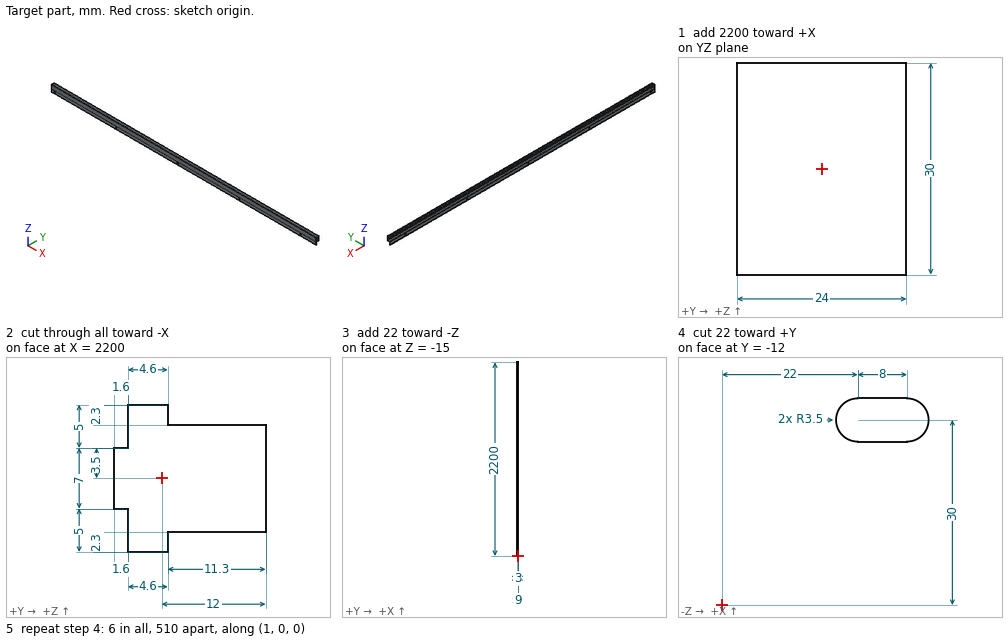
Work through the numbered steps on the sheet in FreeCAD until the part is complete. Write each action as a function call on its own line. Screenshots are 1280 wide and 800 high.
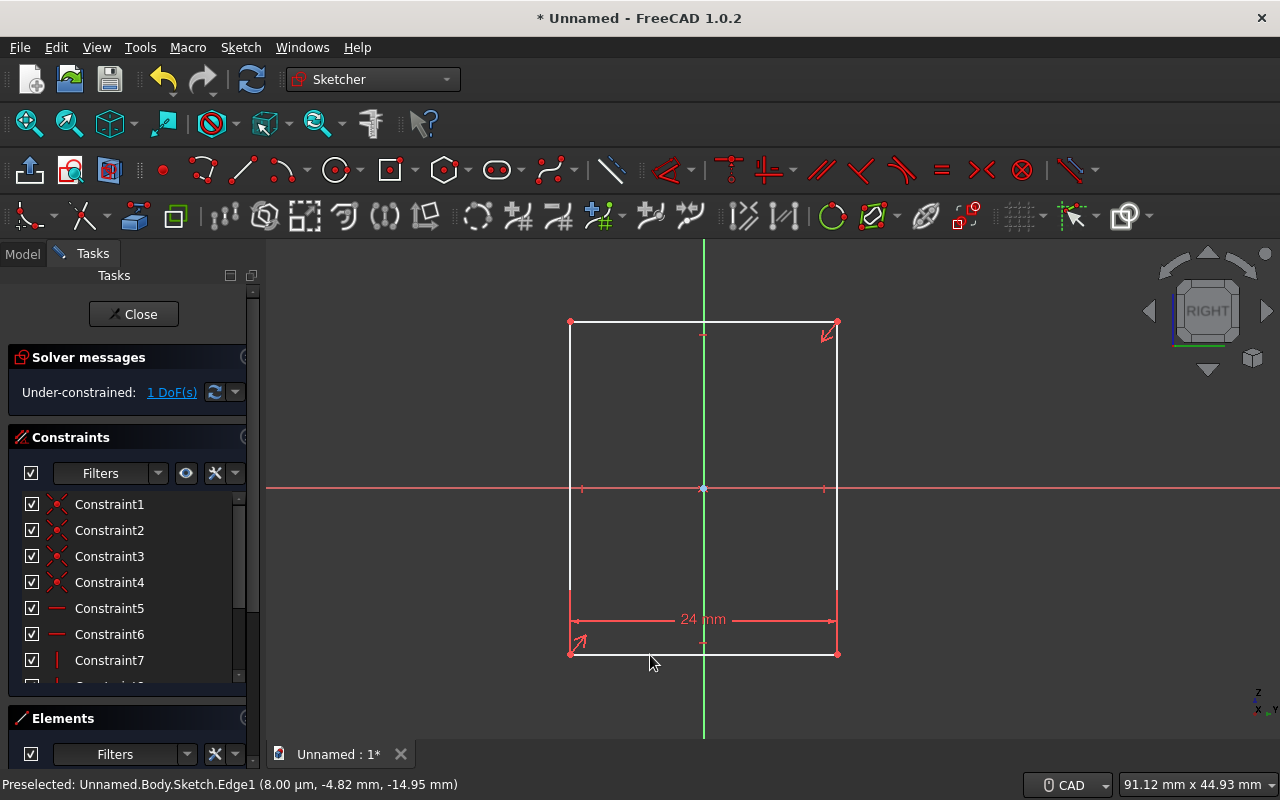
click(837, 555)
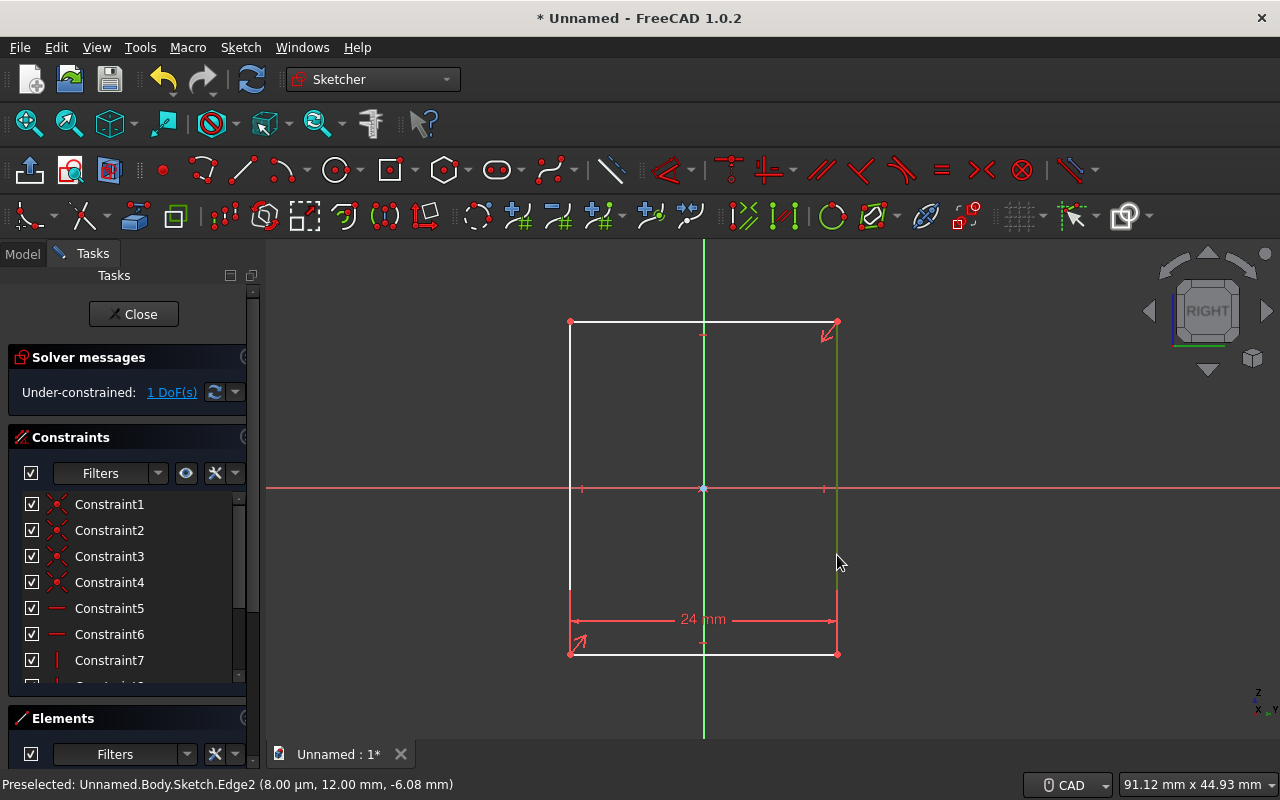
click(694, 170)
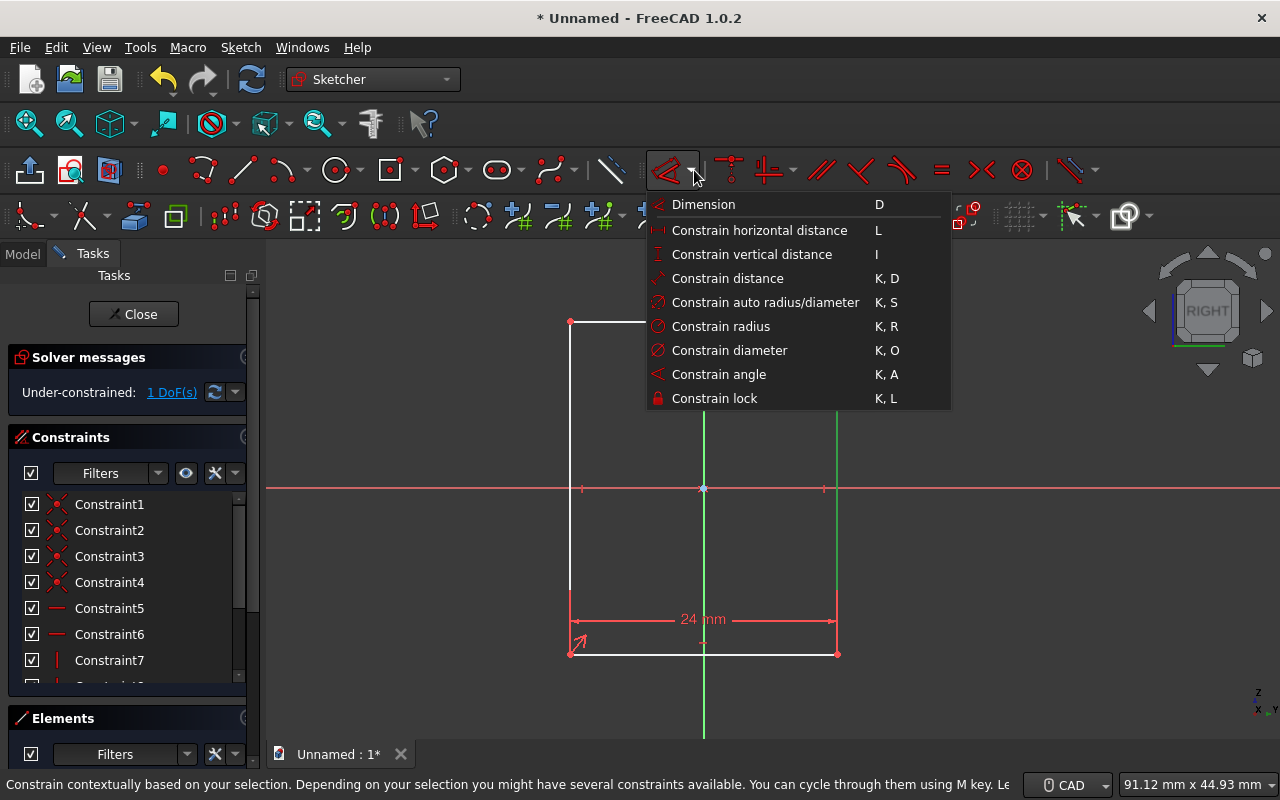
click(799, 254)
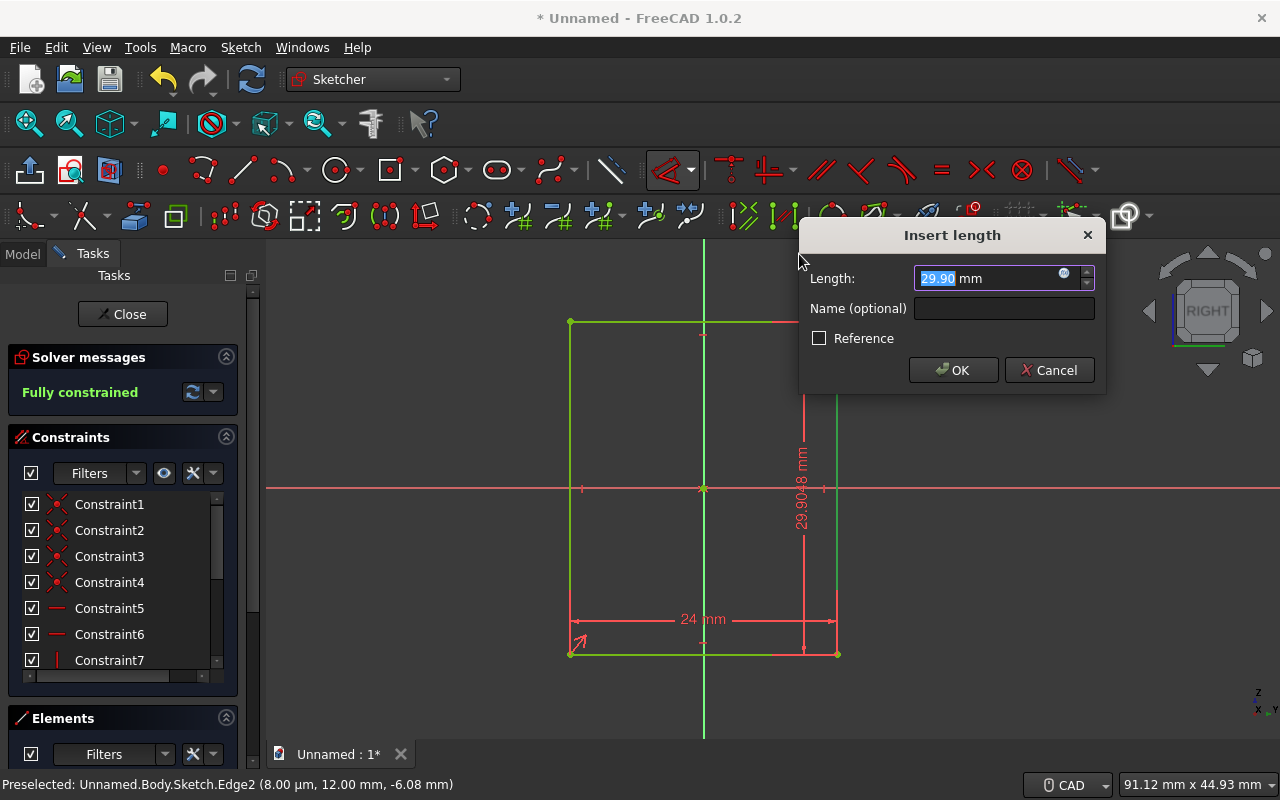
text(30)
key(Return)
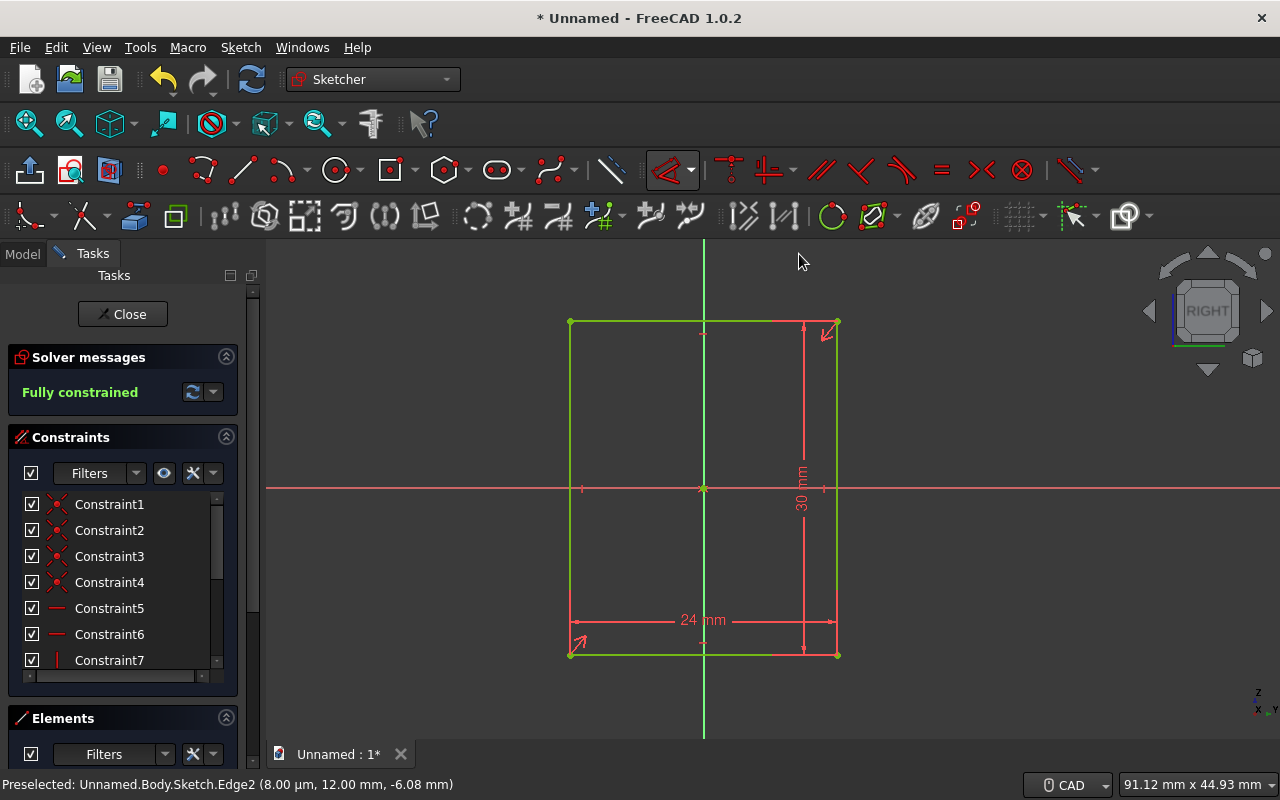
click(123, 314)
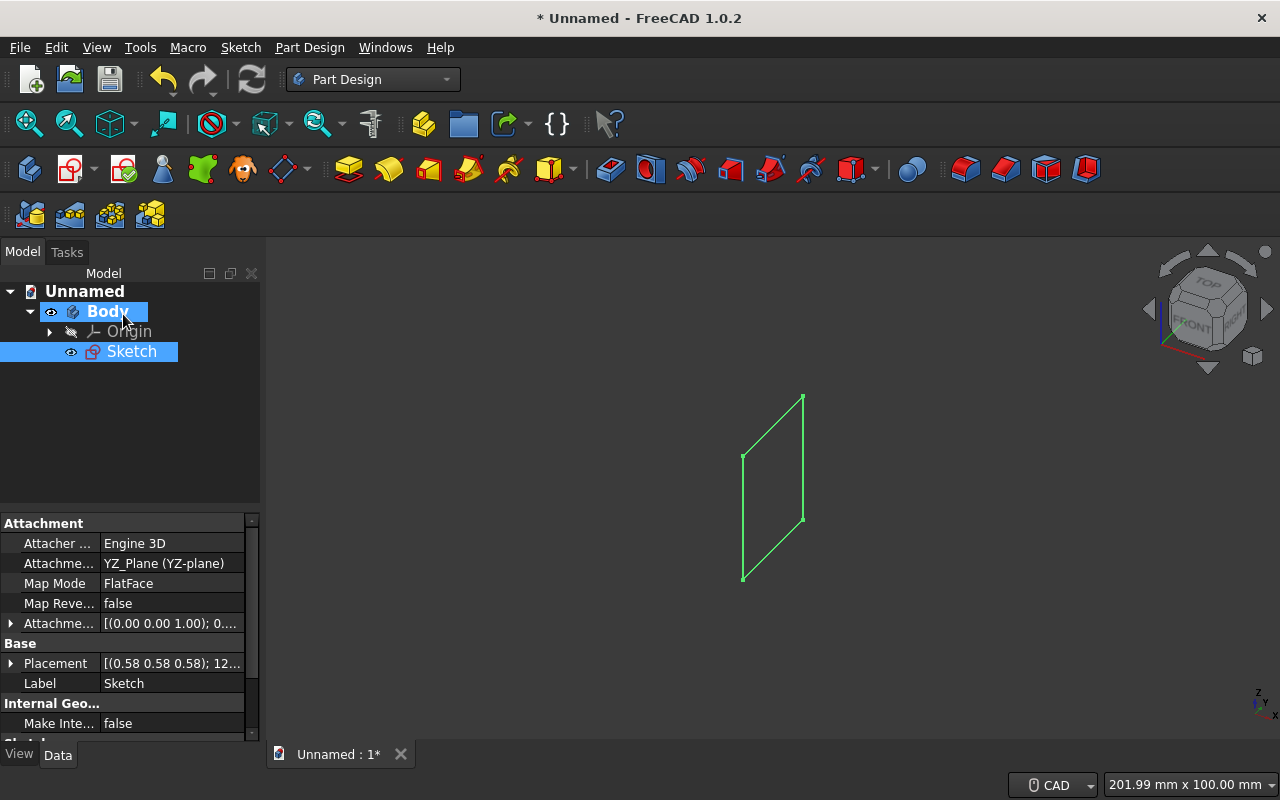
click(350, 170)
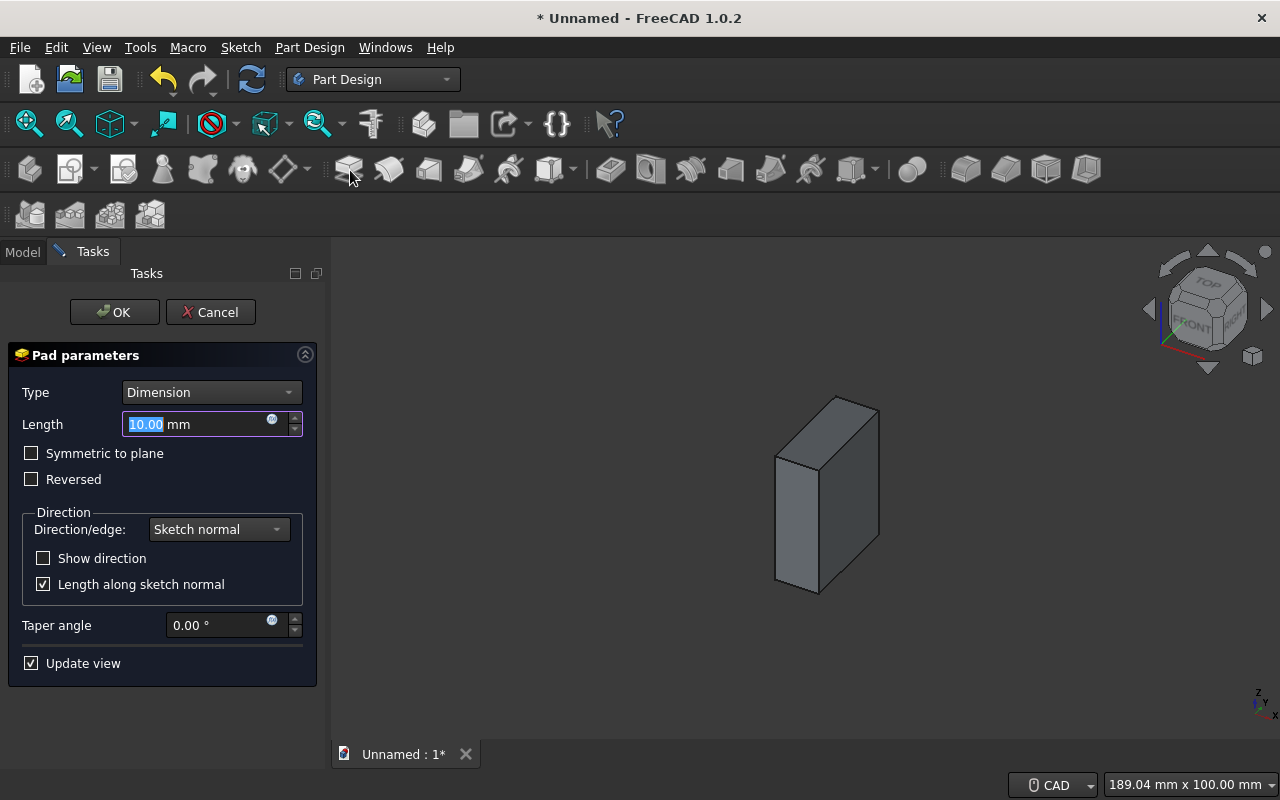
text(2200)
key(Tab)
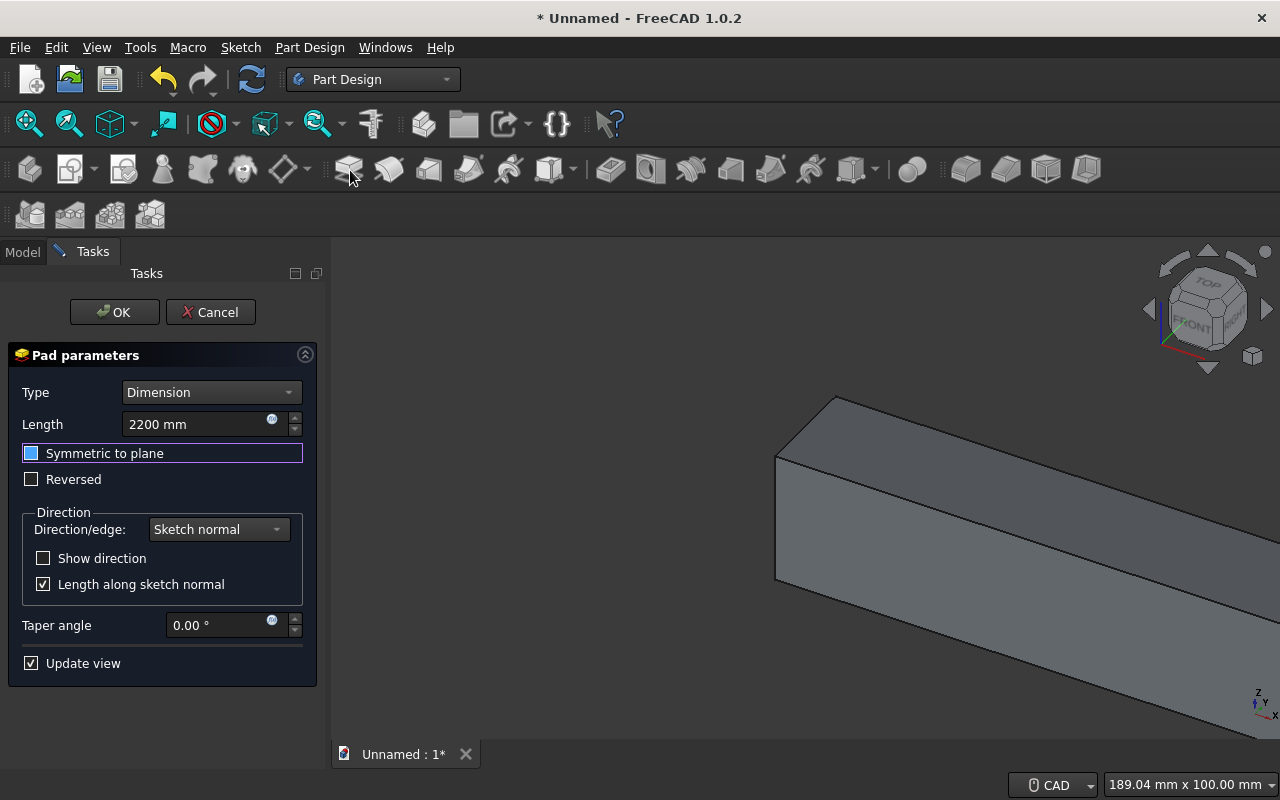
click(115, 312)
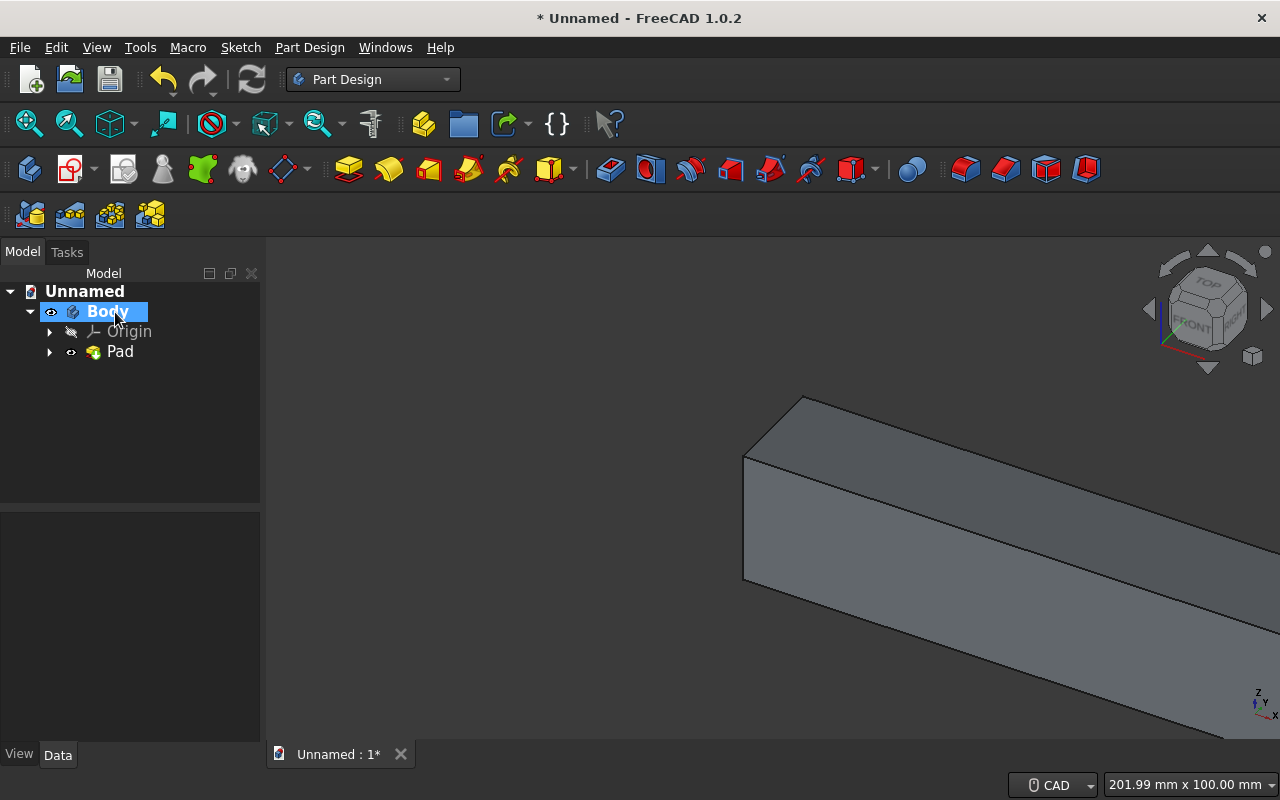
click(30, 124)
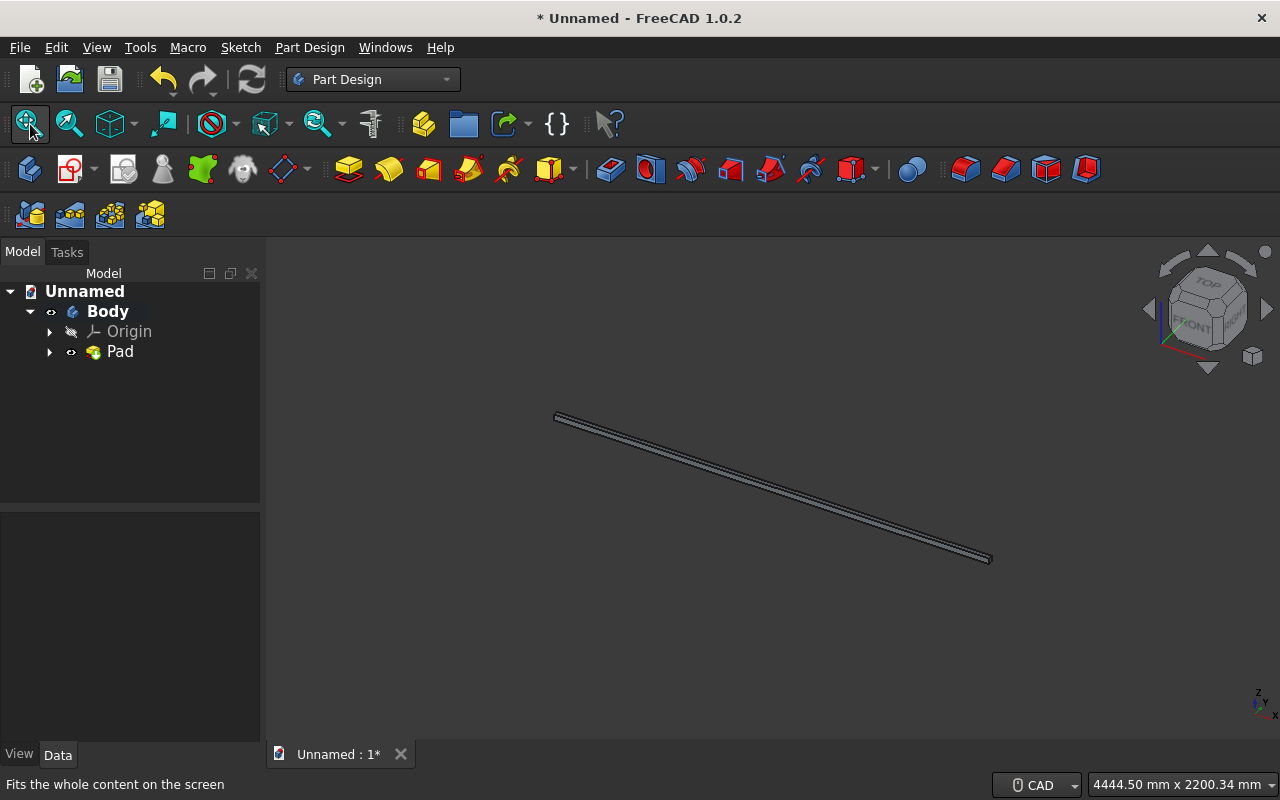
scroll(990, 559, up, 8)